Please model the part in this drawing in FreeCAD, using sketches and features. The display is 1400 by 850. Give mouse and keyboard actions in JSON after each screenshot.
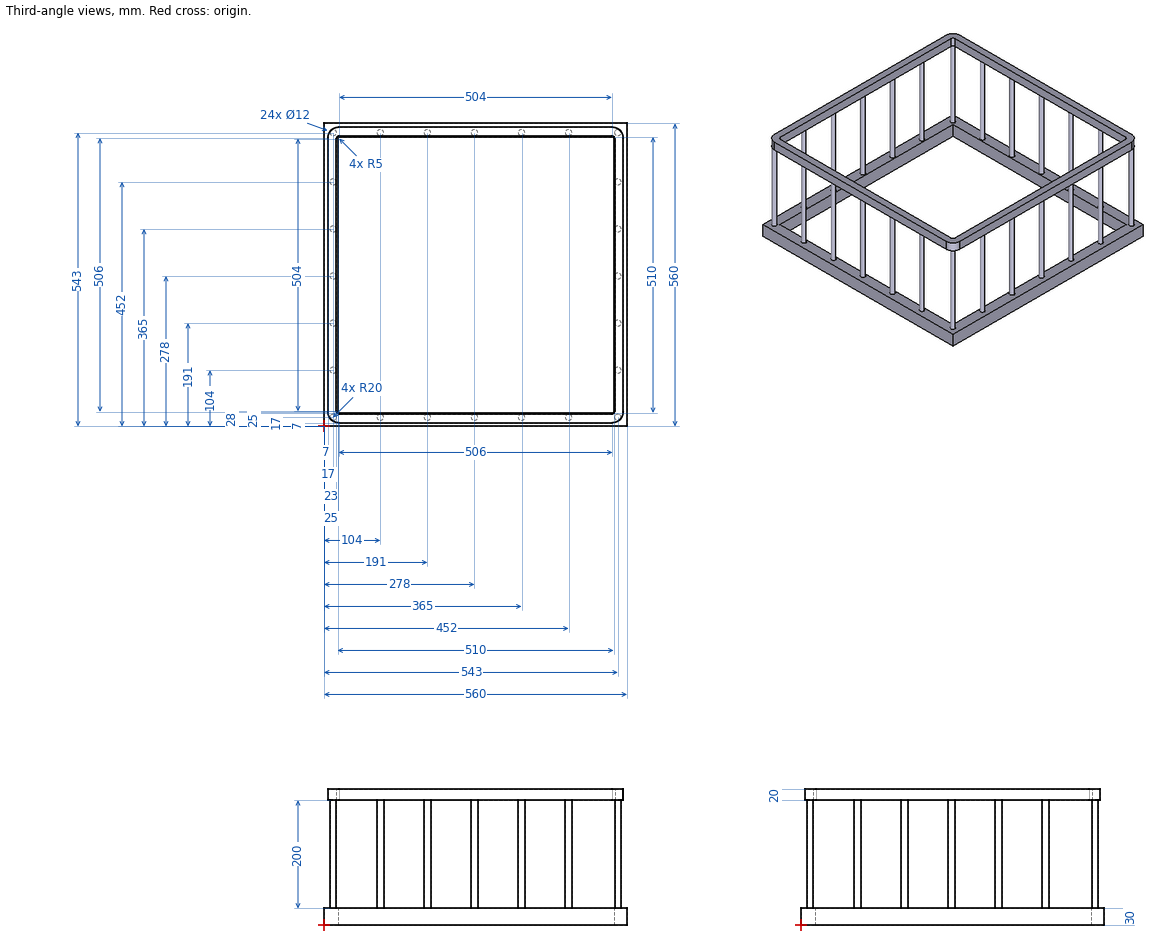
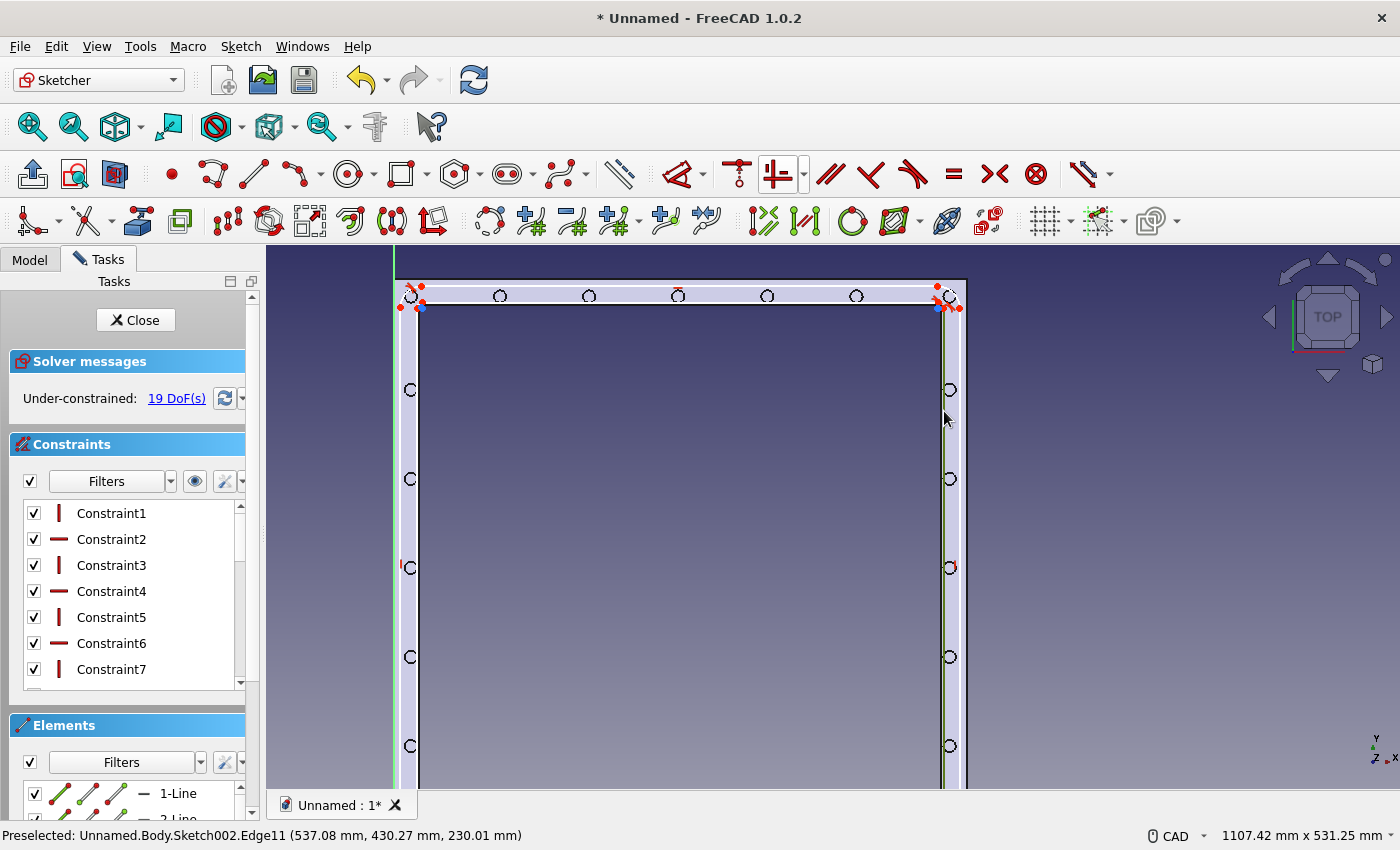
{"action": "scroll", "coordinate": [943, 410], "scroll_direction": "down", "scroll_amount": 2}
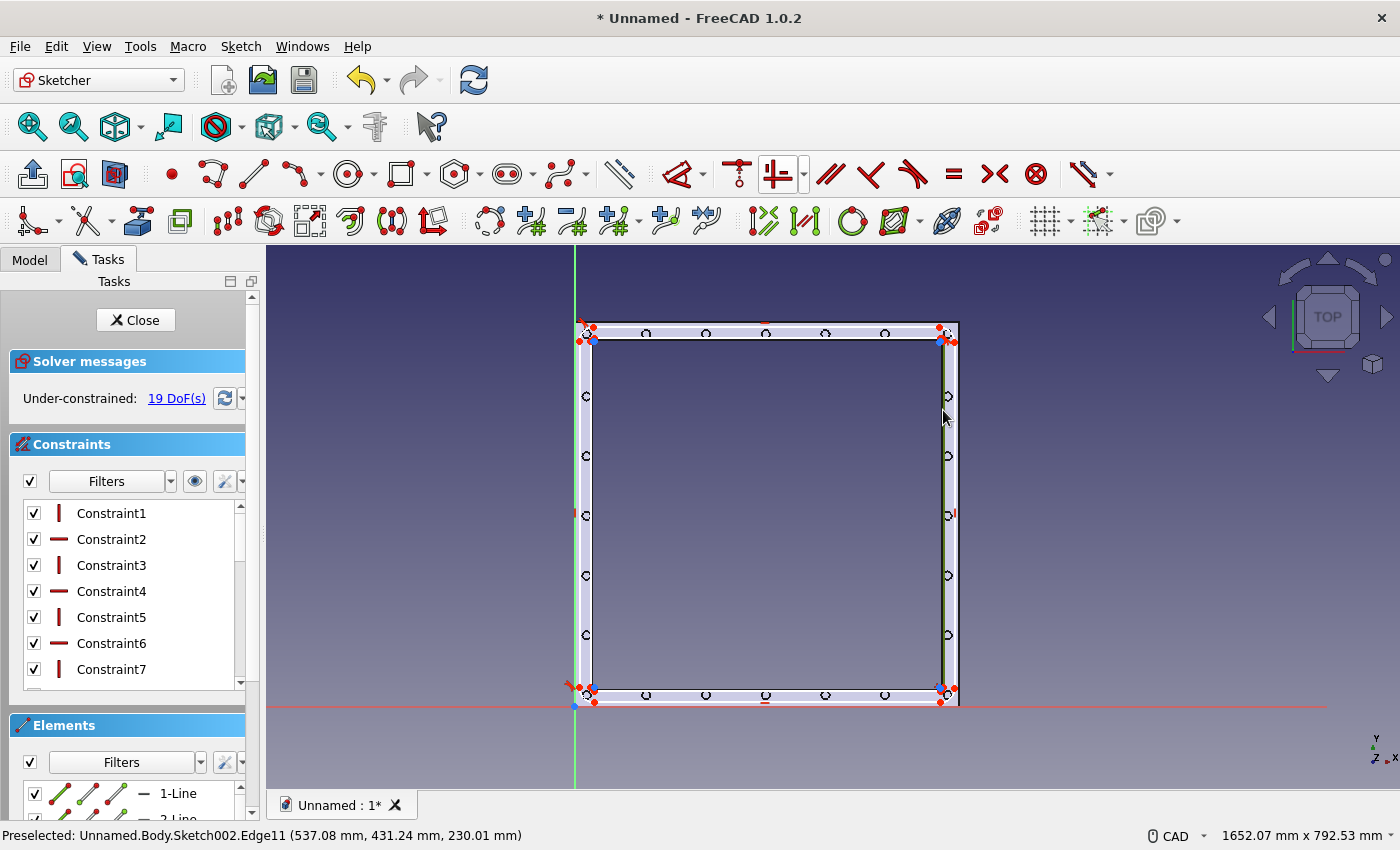
{"action": "scroll", "coordinate": [942, 690], "scroll_direction": "up", "scroll_amount": 9}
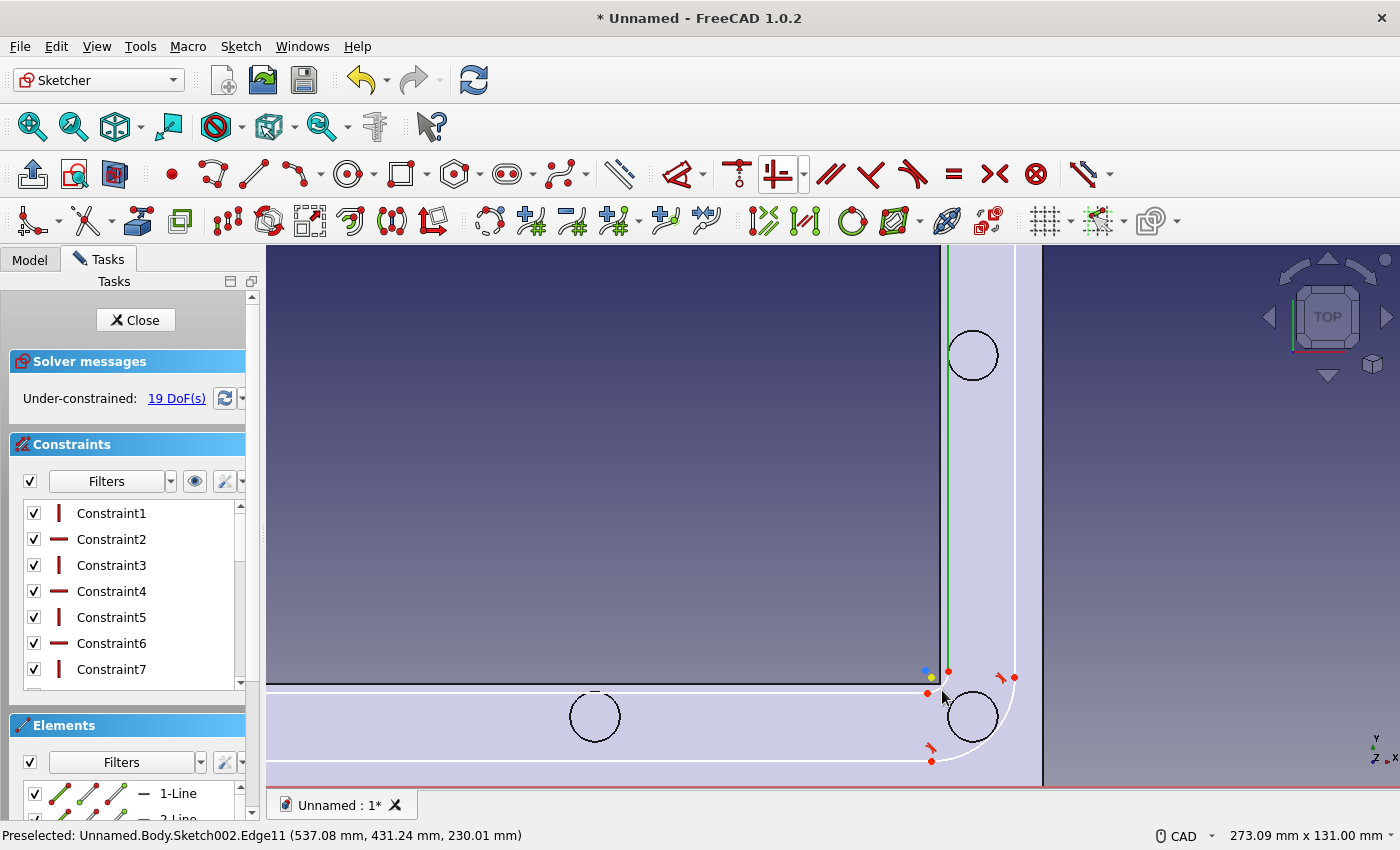
{"action": "left_click", "coordinate": [942, 686]}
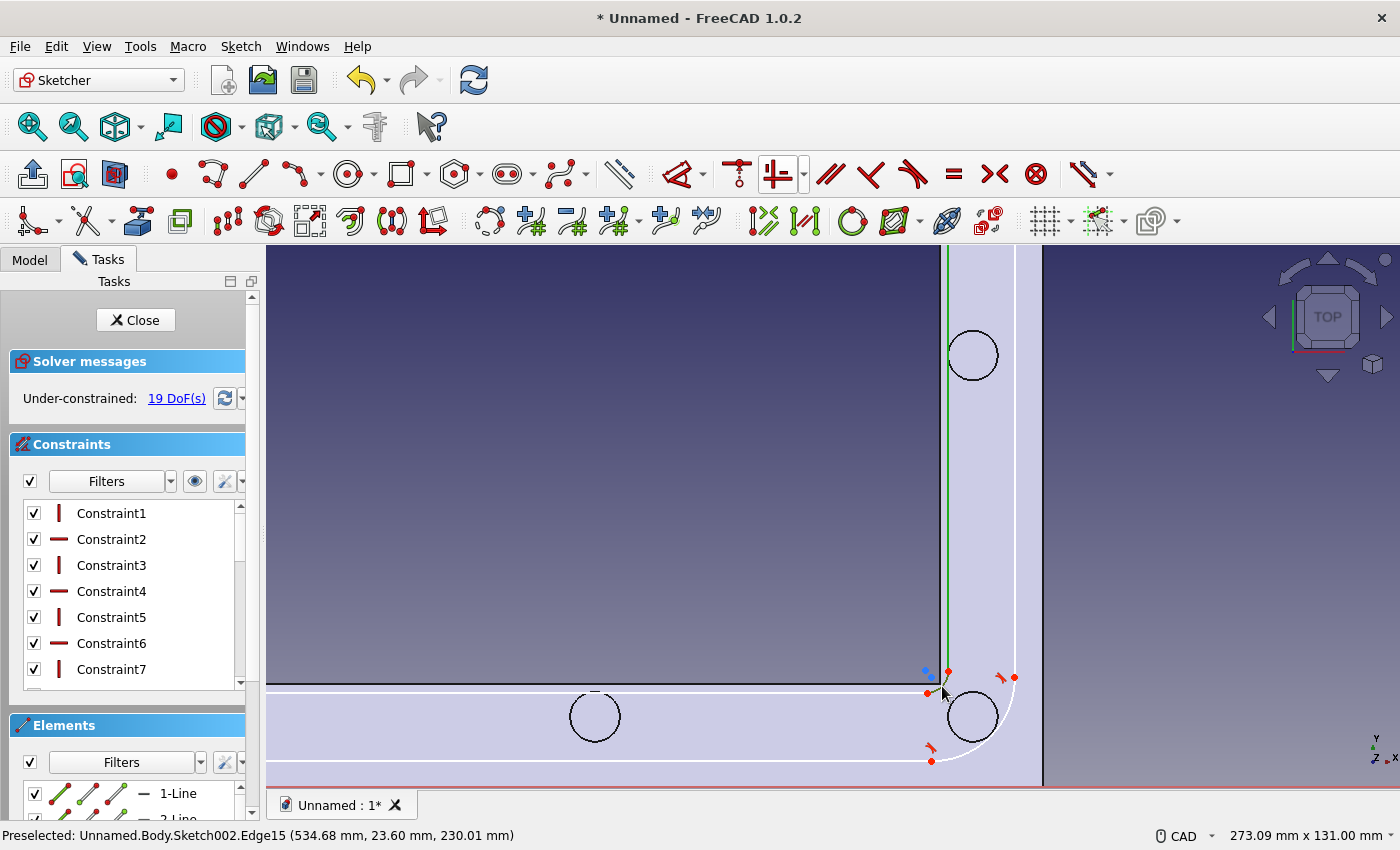
{"action": "left_click", "coordinate": [913, 174]}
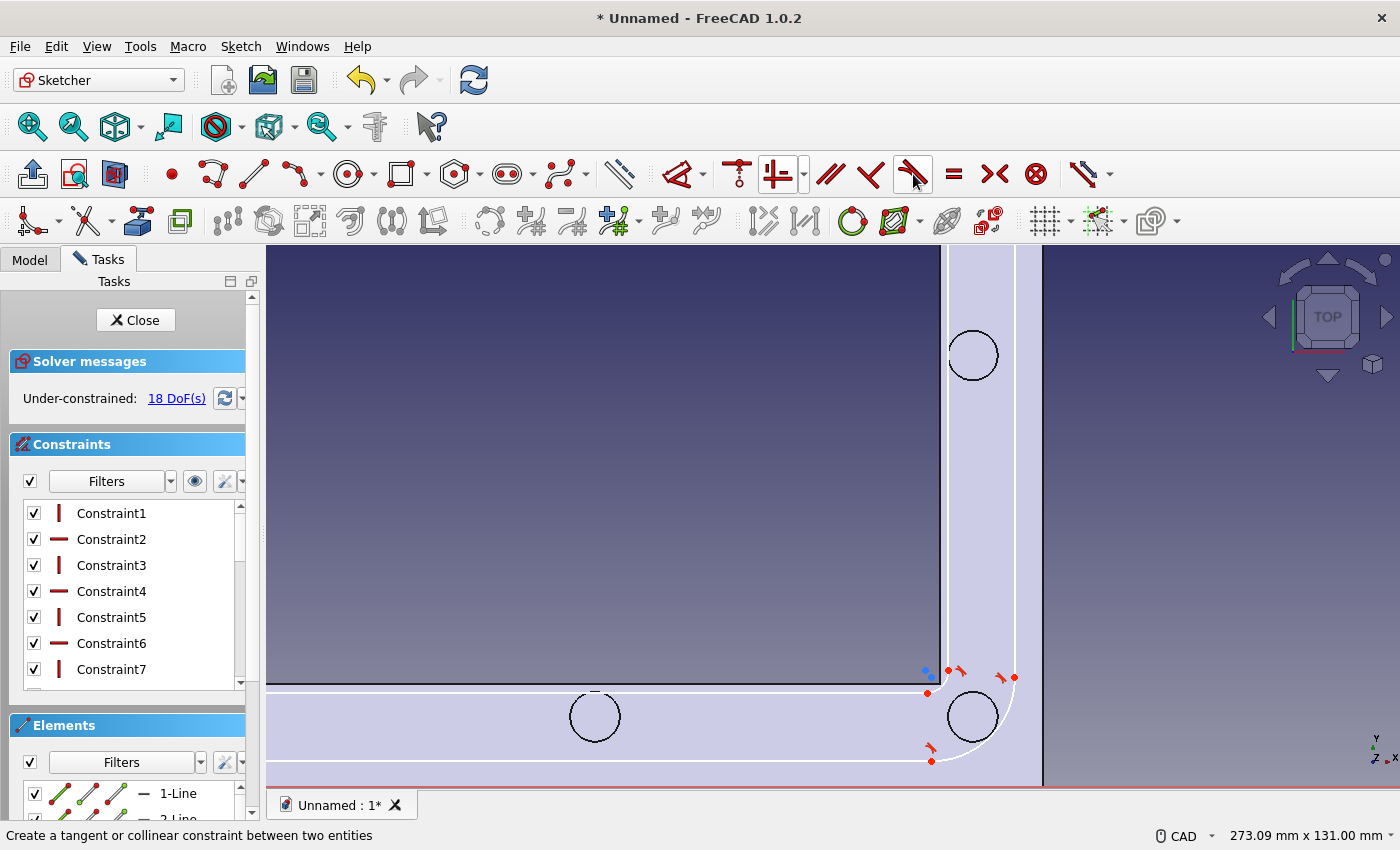
{"action": "scroll", "coordinate": [942, 691], "scroll_direction": "down", "scroll_amount": 9}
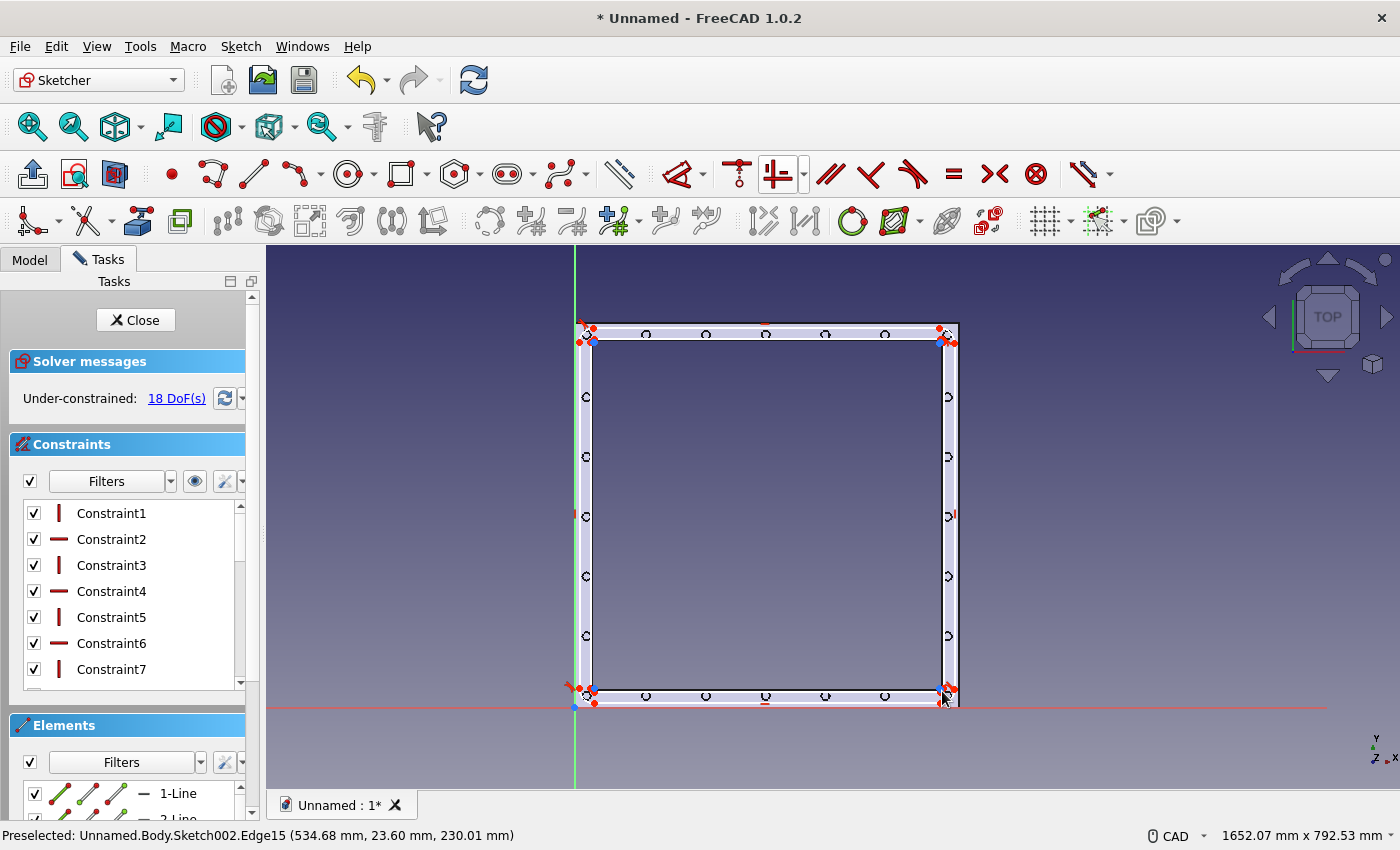
{"action": "scroll", "coordinate": [836, 692], "scroll_direction": "up", "scroll_amount": 2}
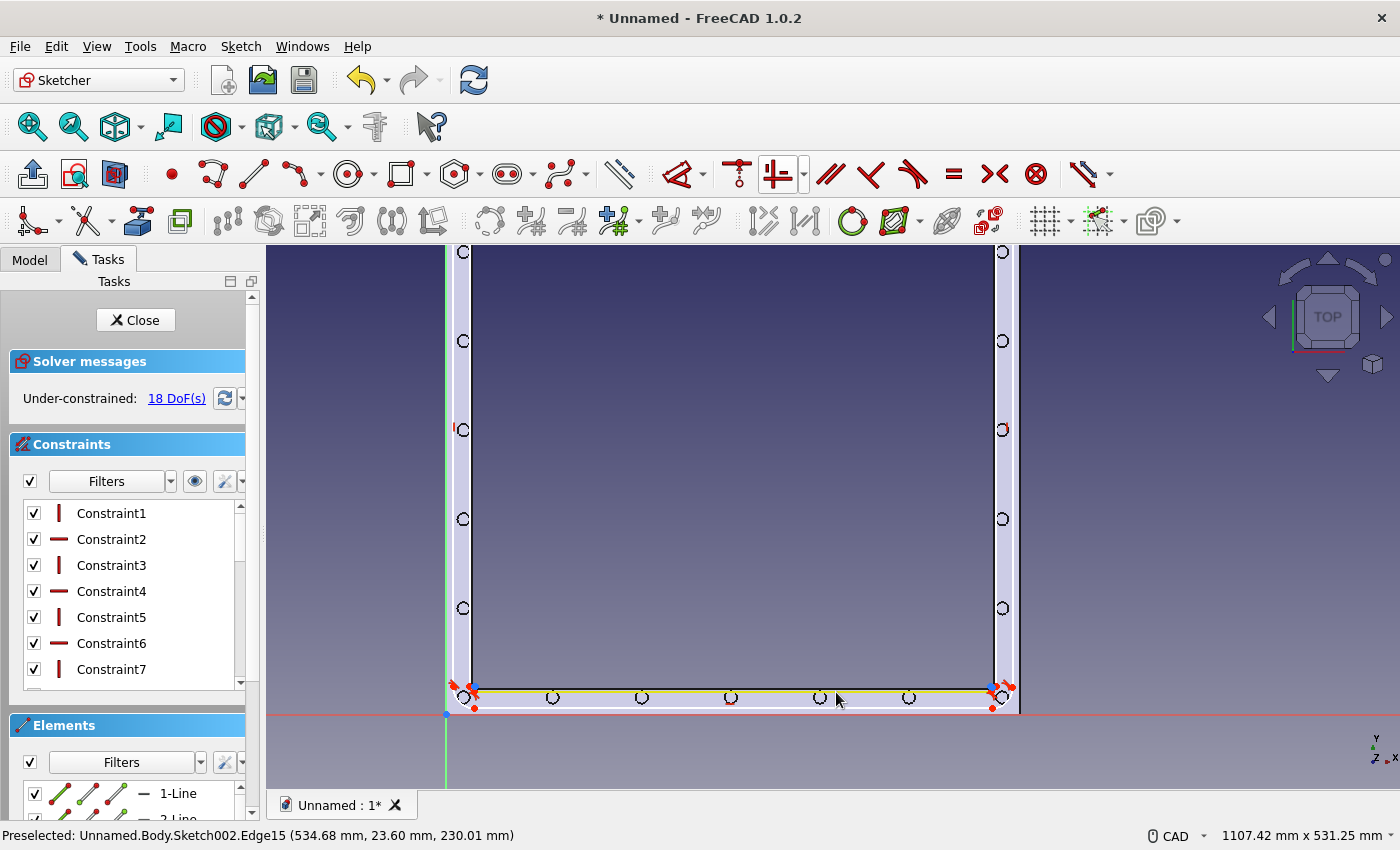
{"action": "left_click", "coordinate": [836, 692]}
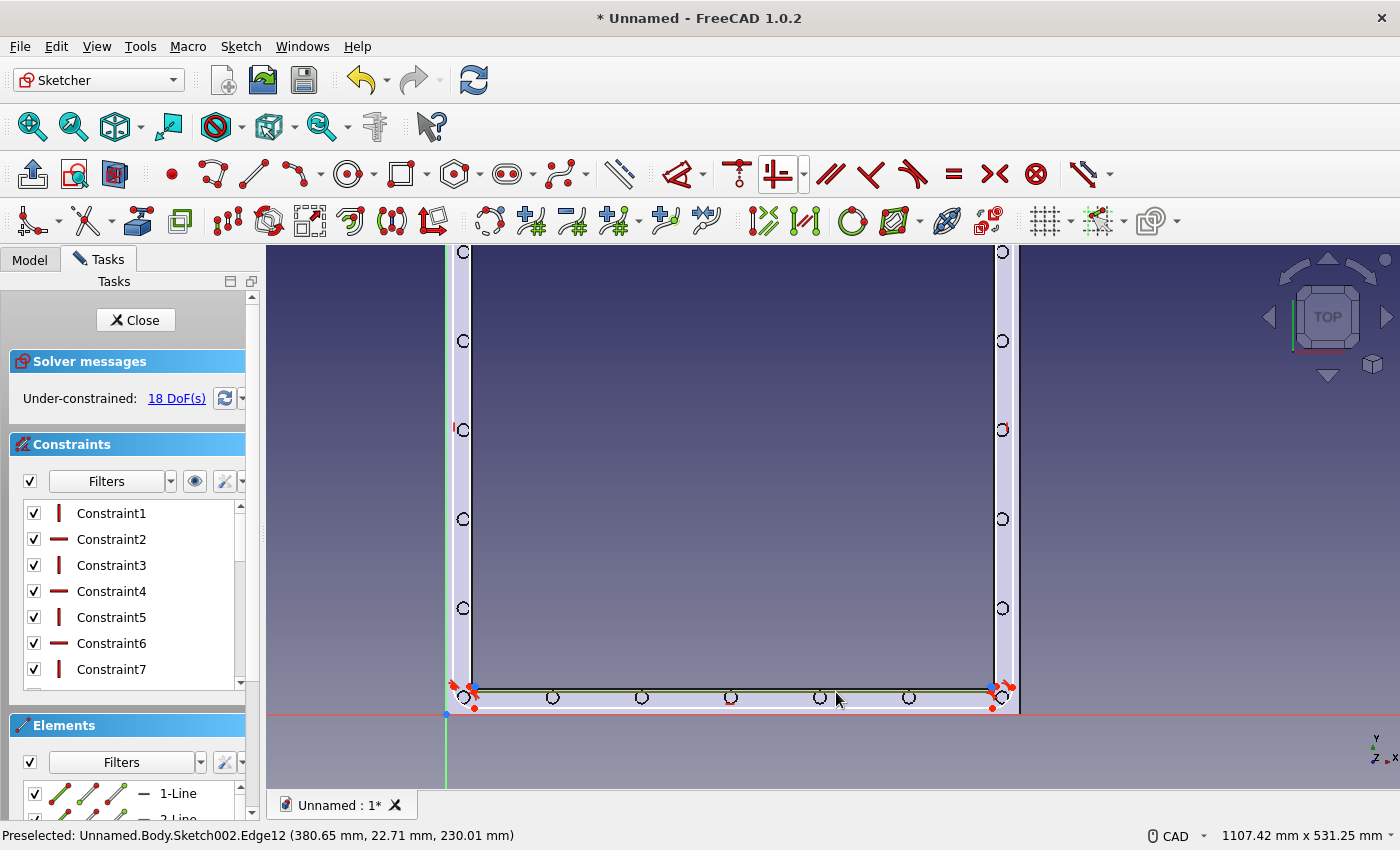
{"action": "scroll", "coordinate": [995, 690], "scroll_direction": "up", "scroll_amount": 7}